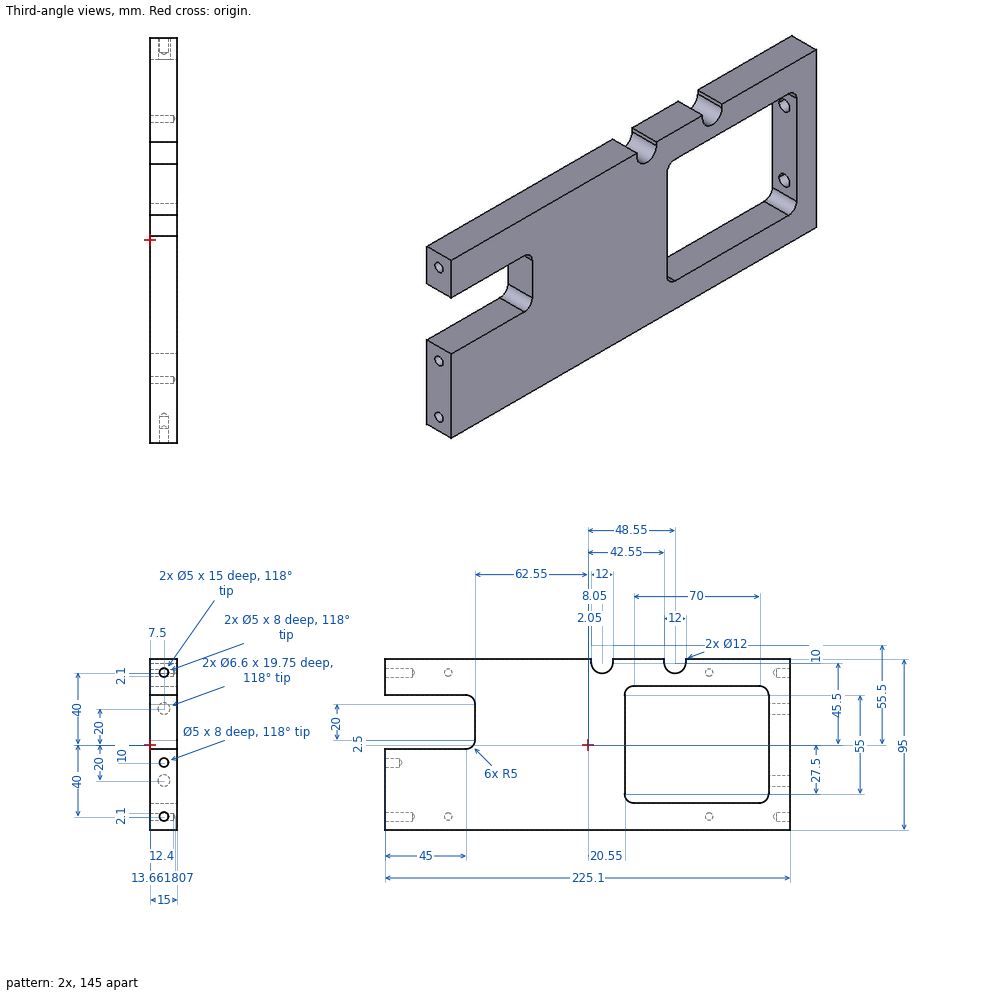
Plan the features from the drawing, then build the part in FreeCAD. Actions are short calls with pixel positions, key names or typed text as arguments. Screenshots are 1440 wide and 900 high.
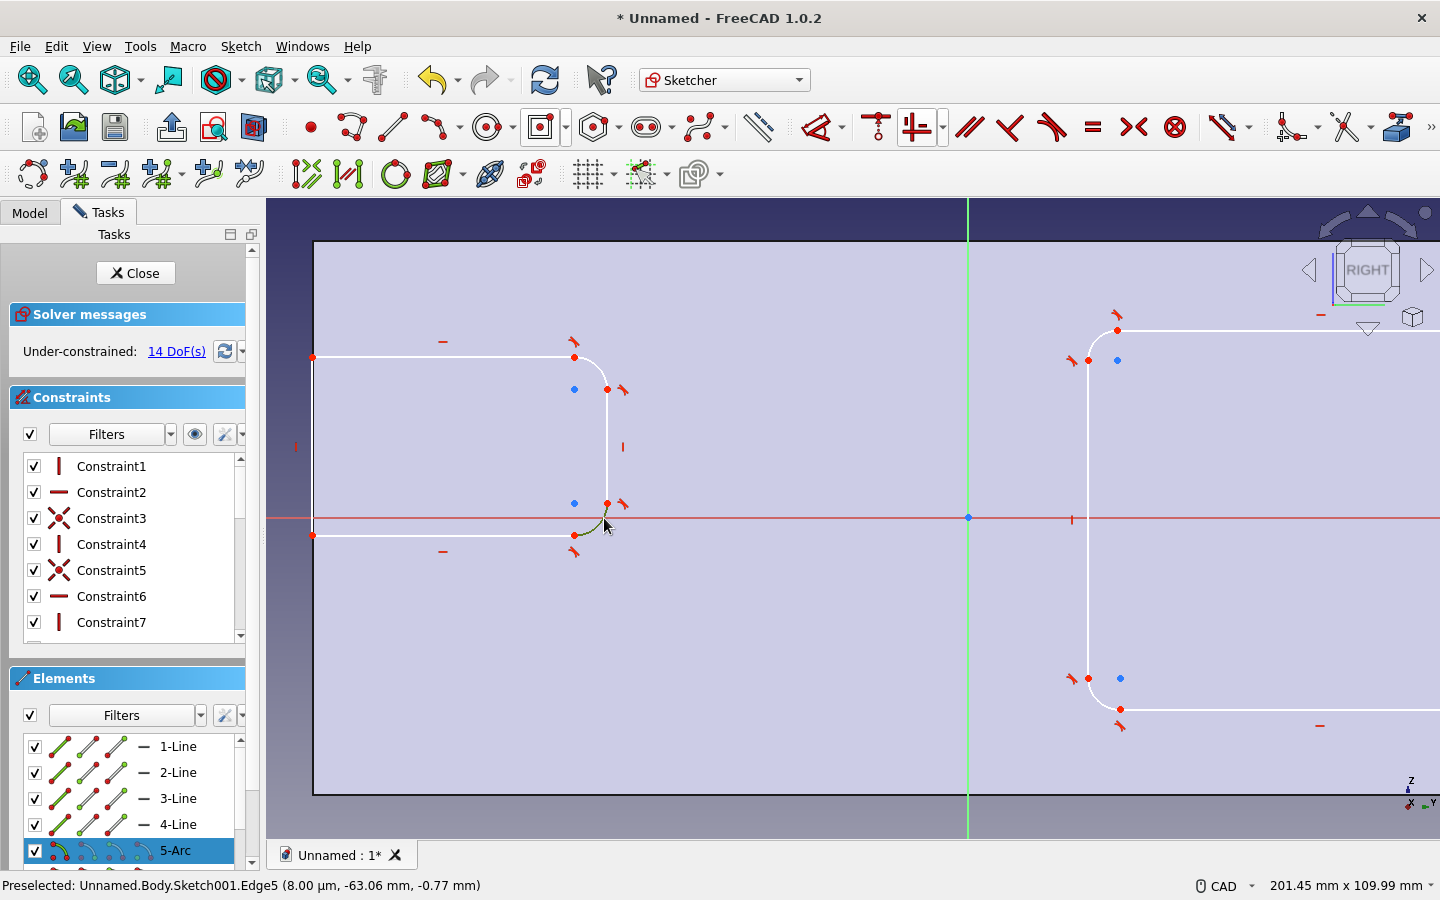
click(604, 375)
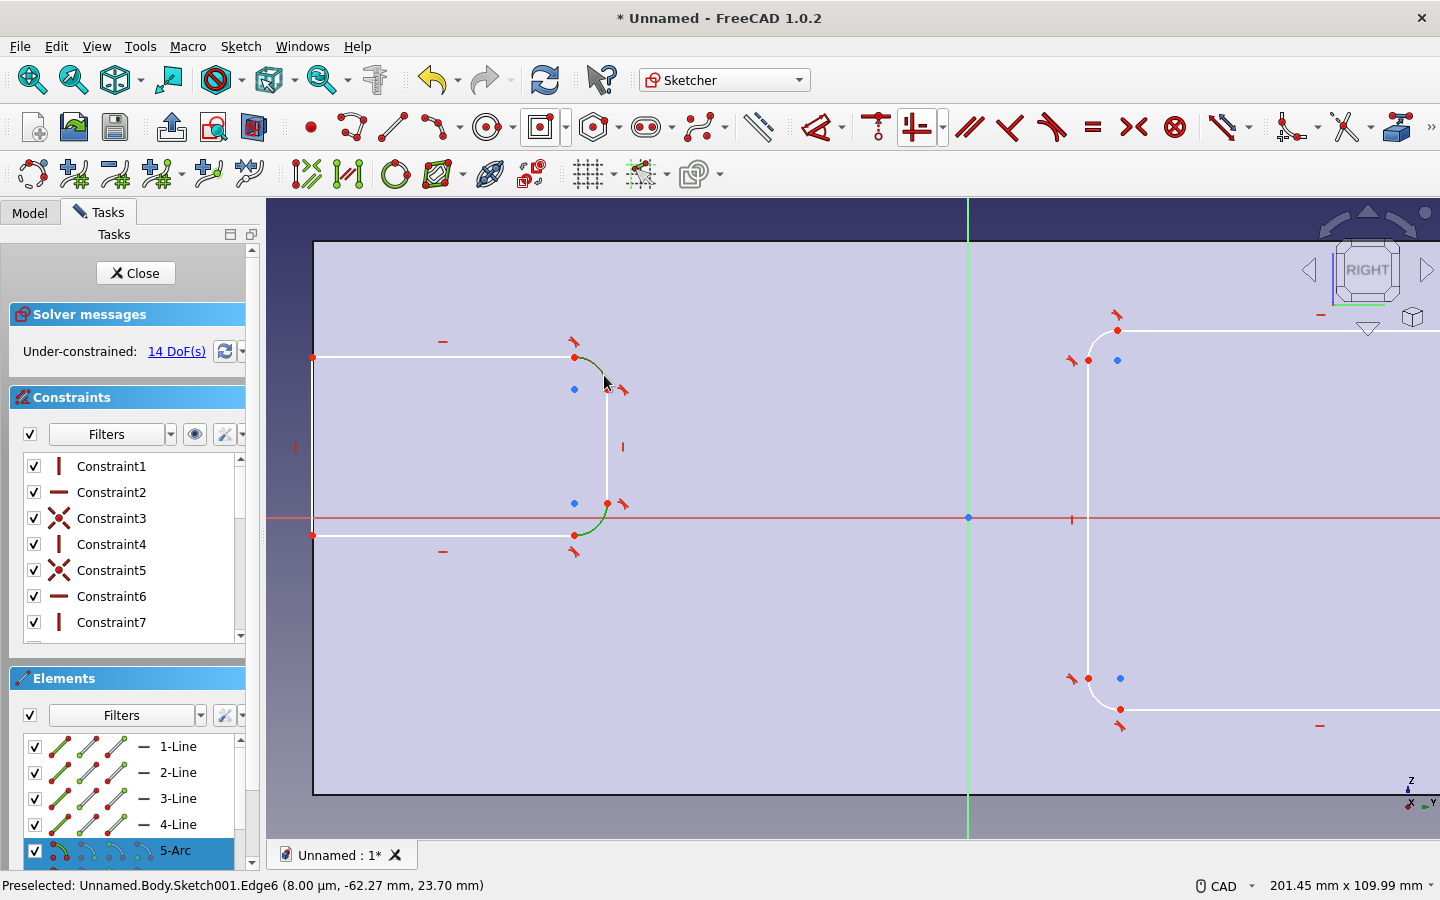
click(1104, 334)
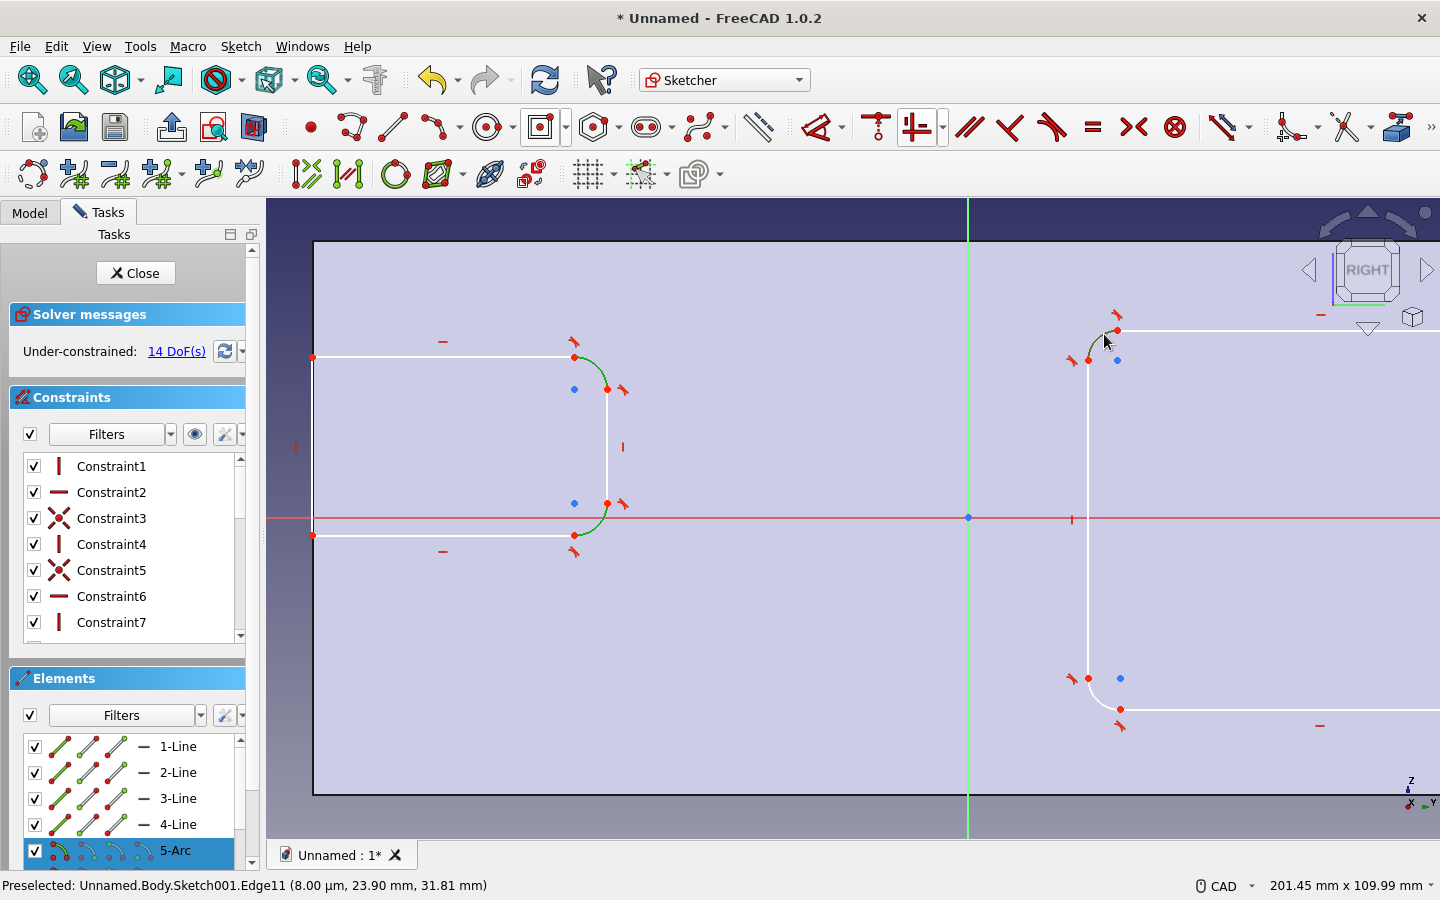
scroll(603, 519, down, 3)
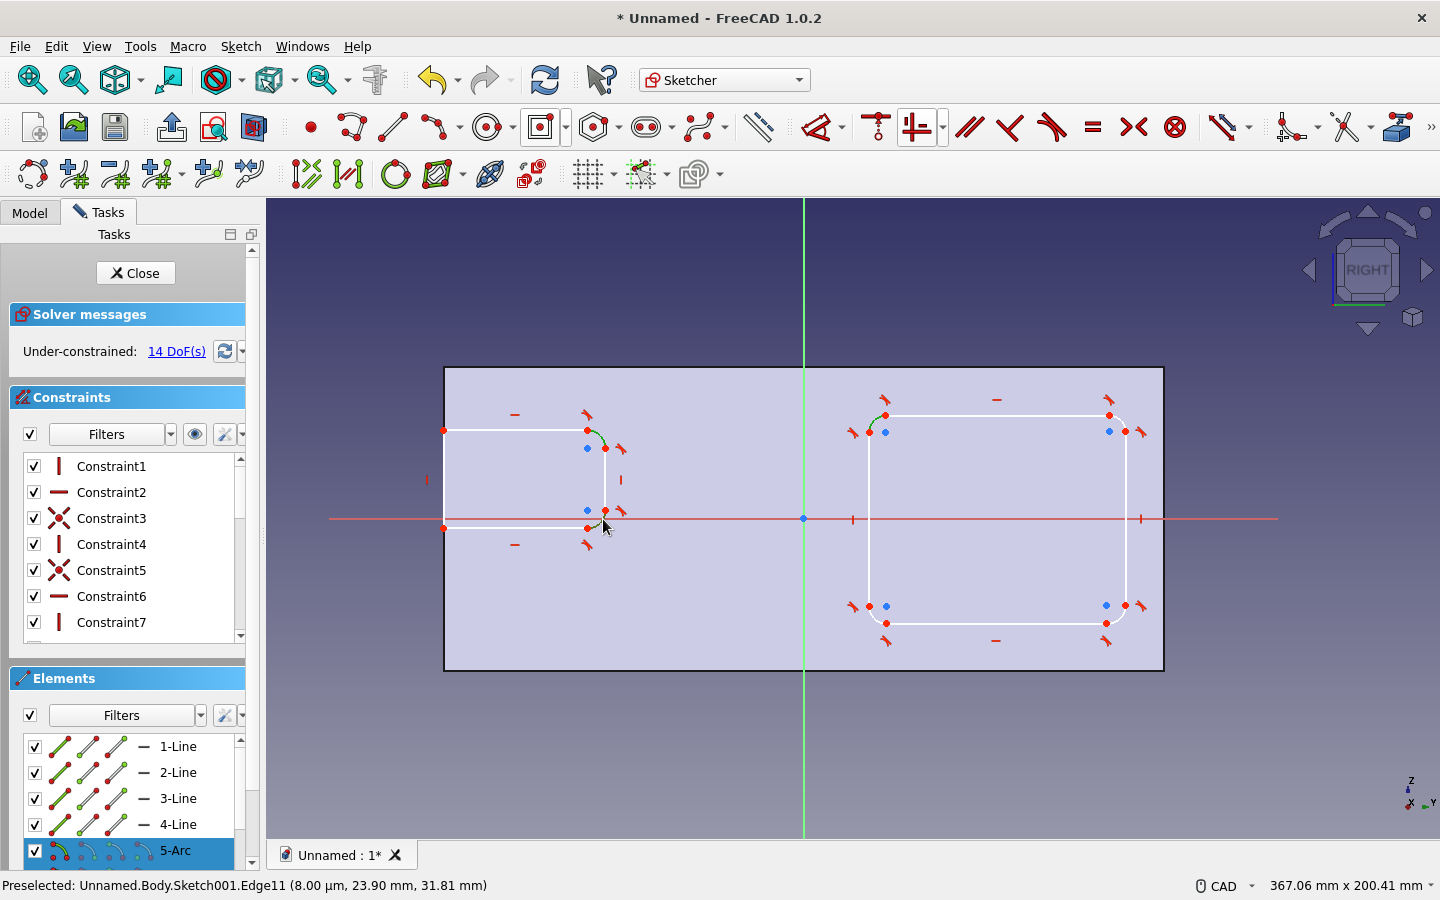
scroll(1124, 425, up, 4)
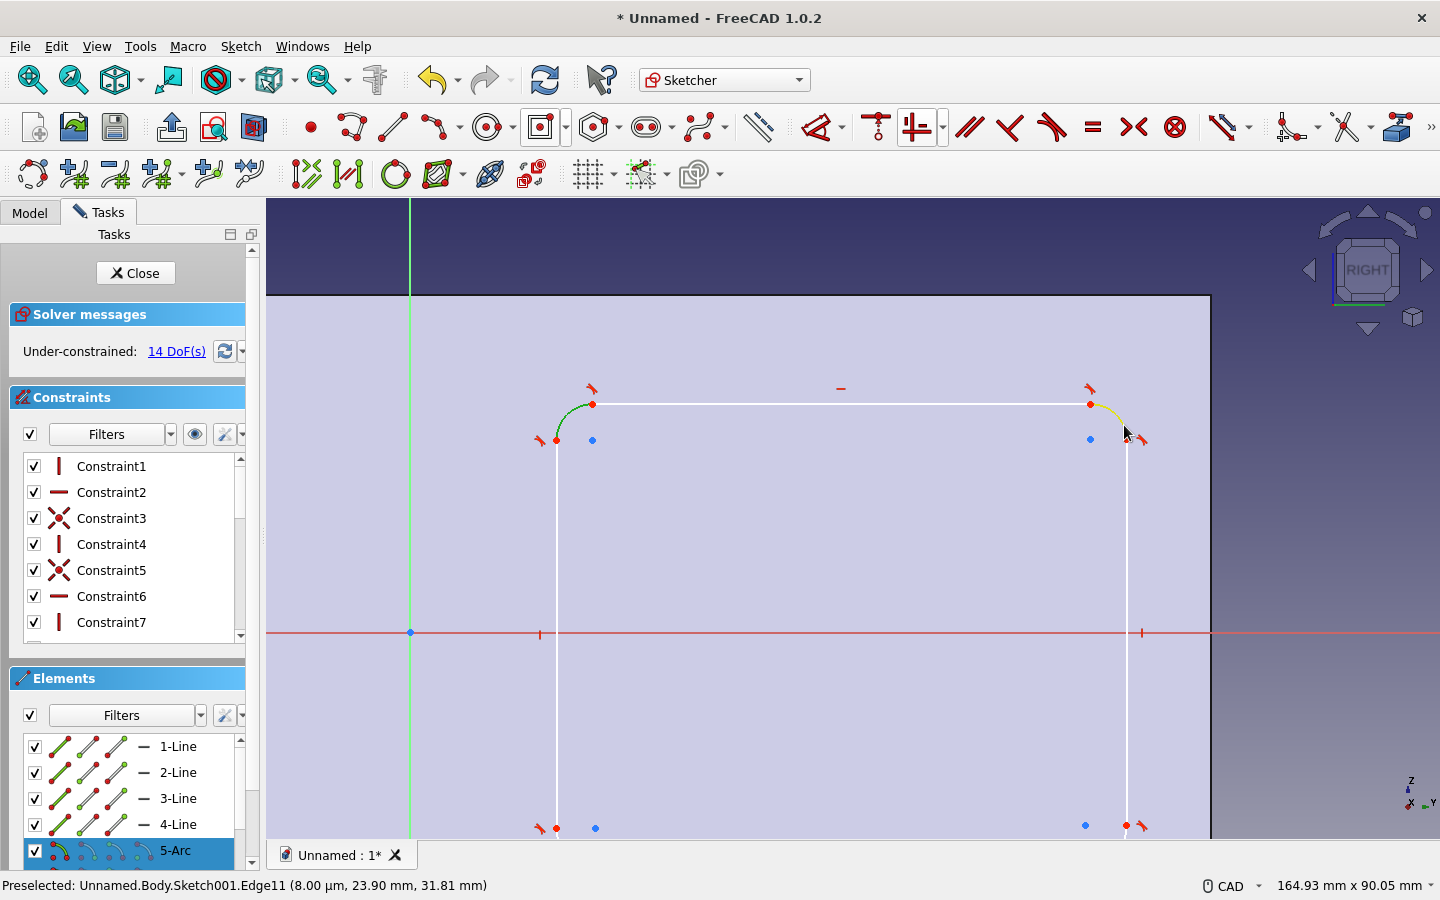
click(1123, 424)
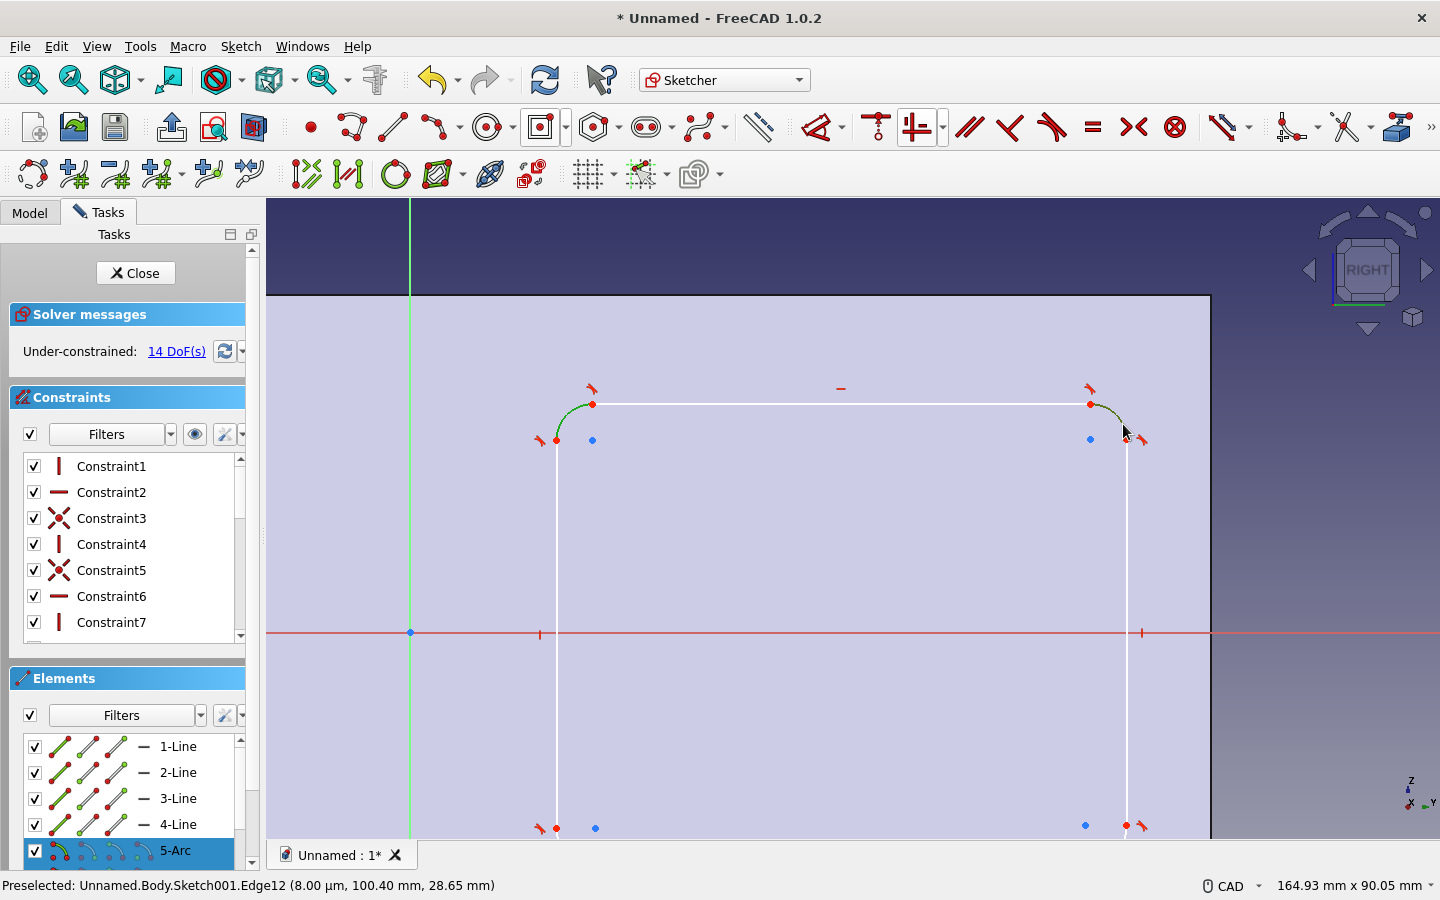
scroll(1125, 425, down, 4)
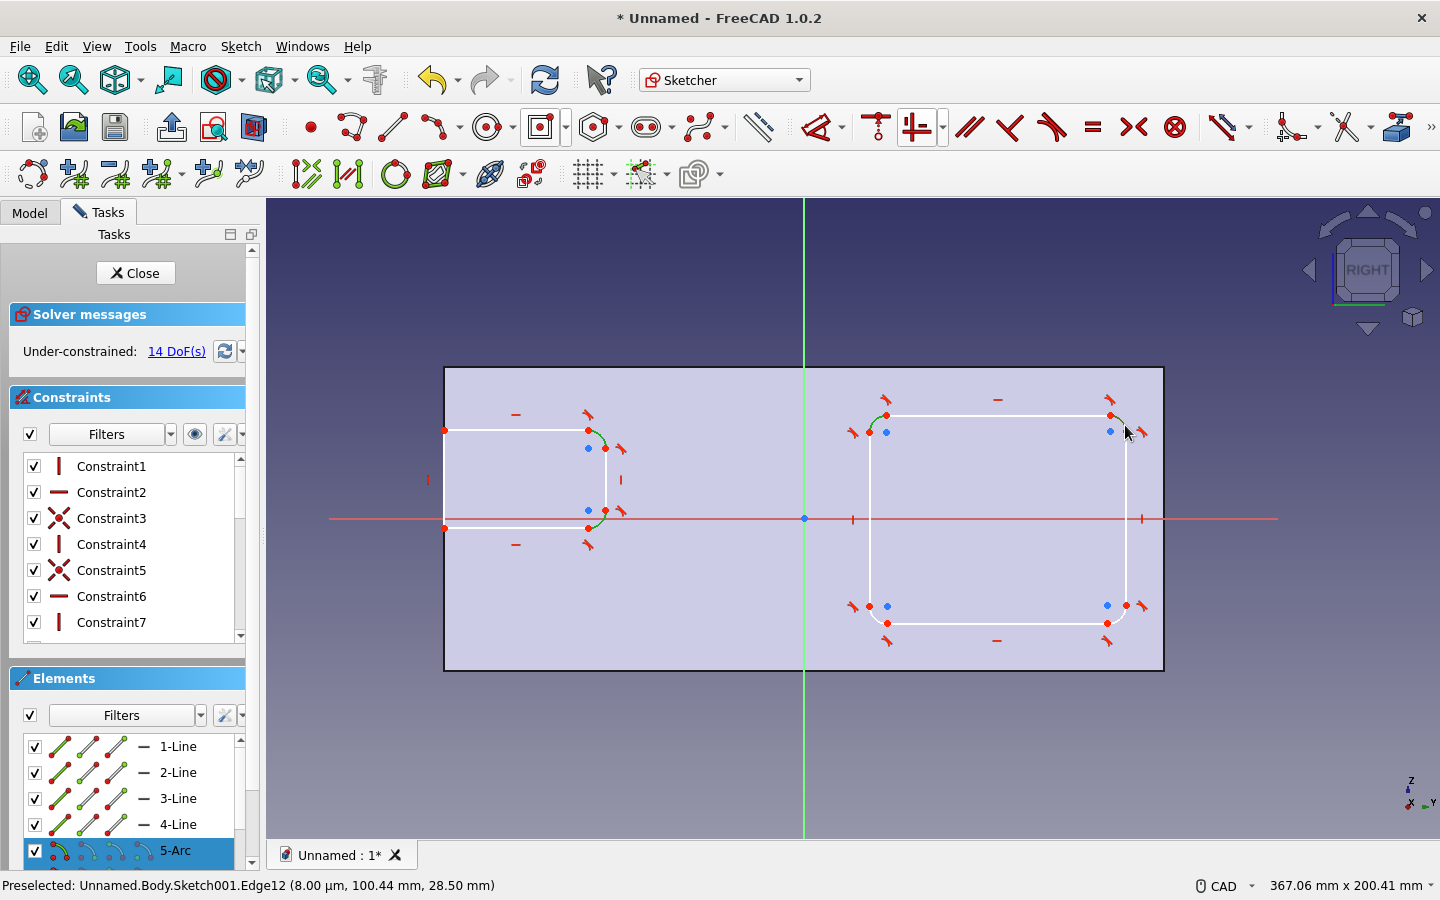
scroll(1116, 622, up, 3)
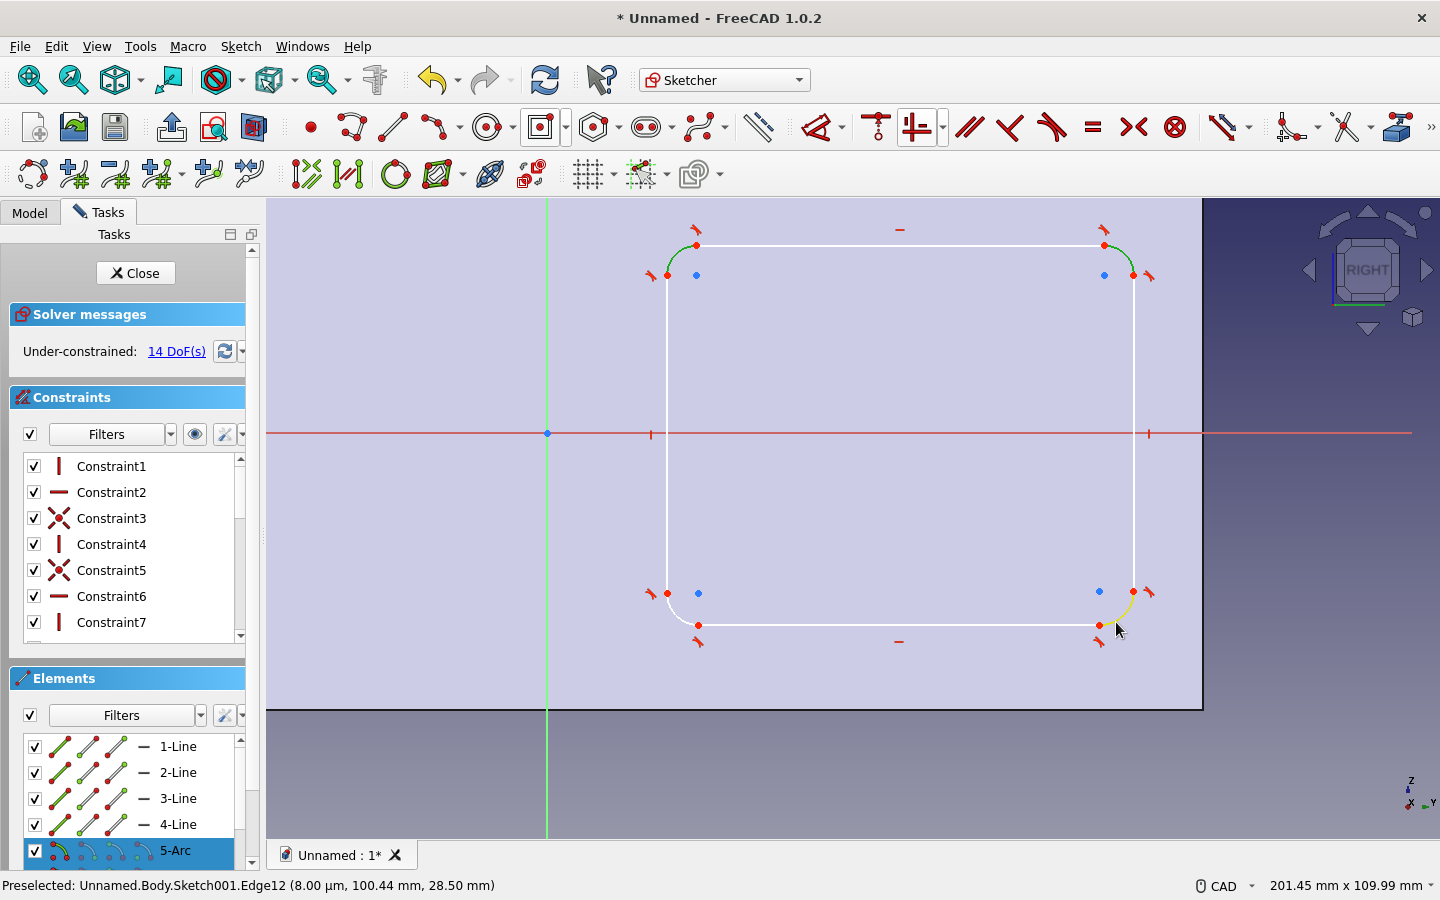
click(1115, 621)